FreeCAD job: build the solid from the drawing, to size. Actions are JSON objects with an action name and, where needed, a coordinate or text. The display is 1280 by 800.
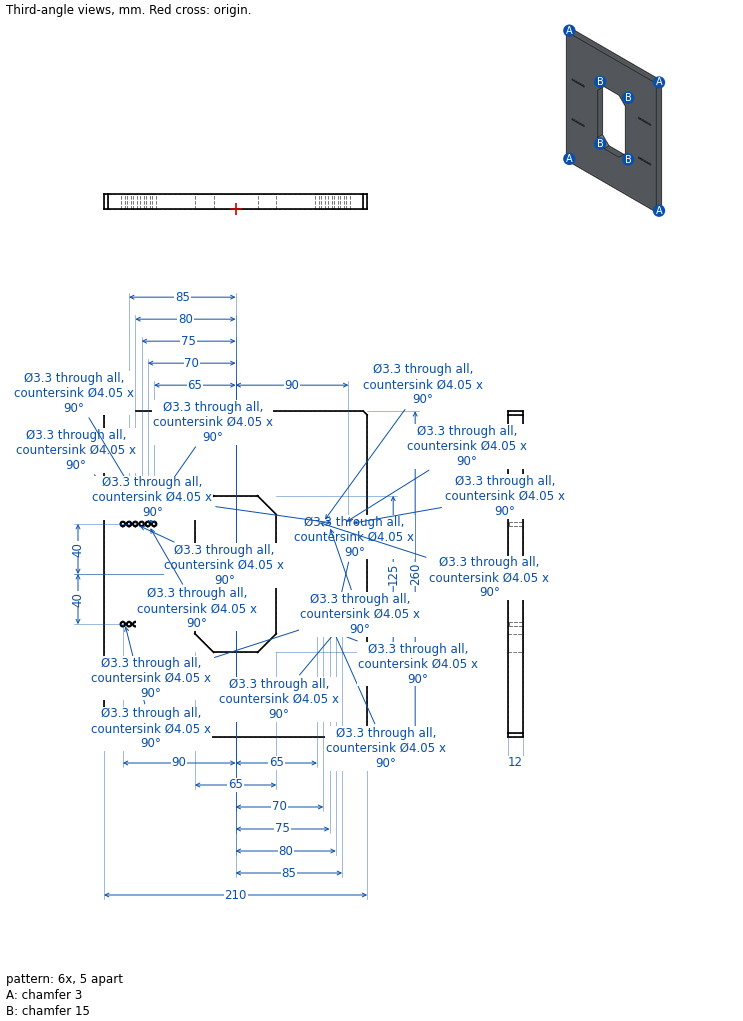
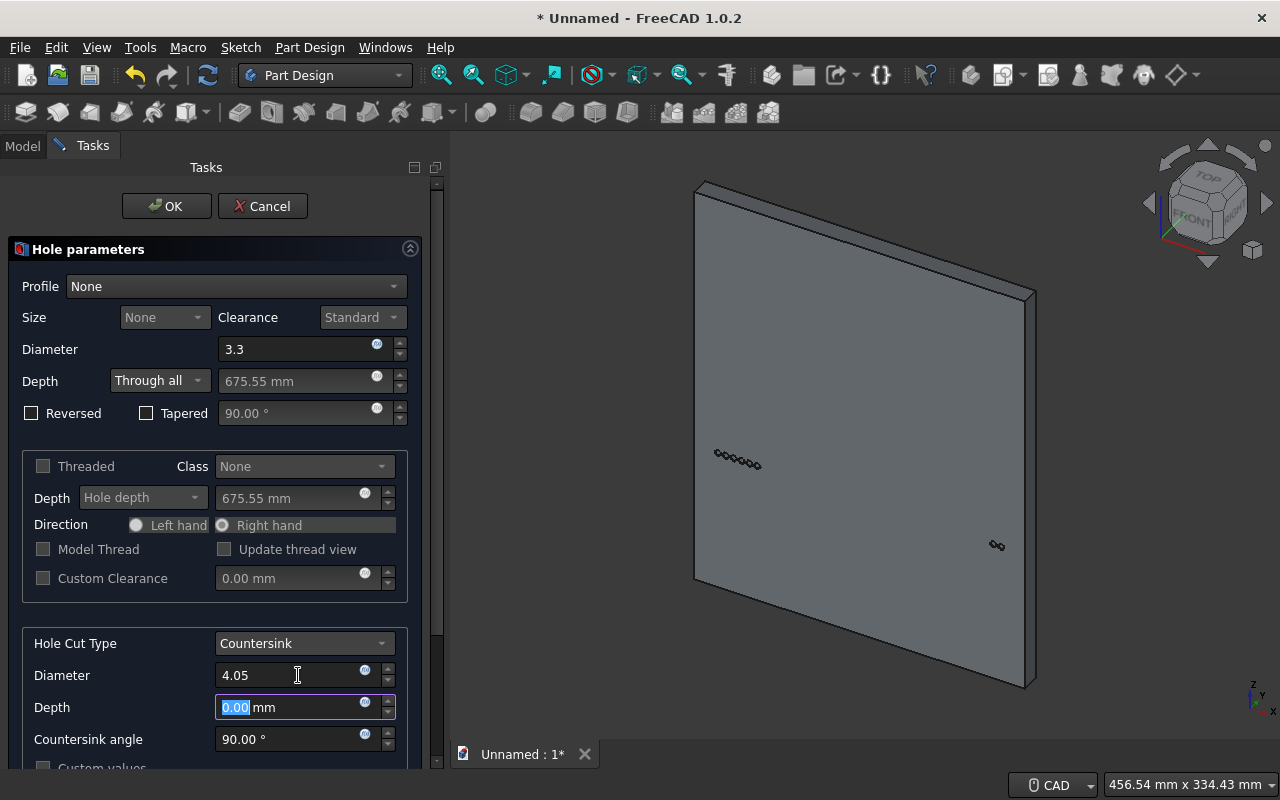
{"action": "left_click", "coordinate": [167, 206]}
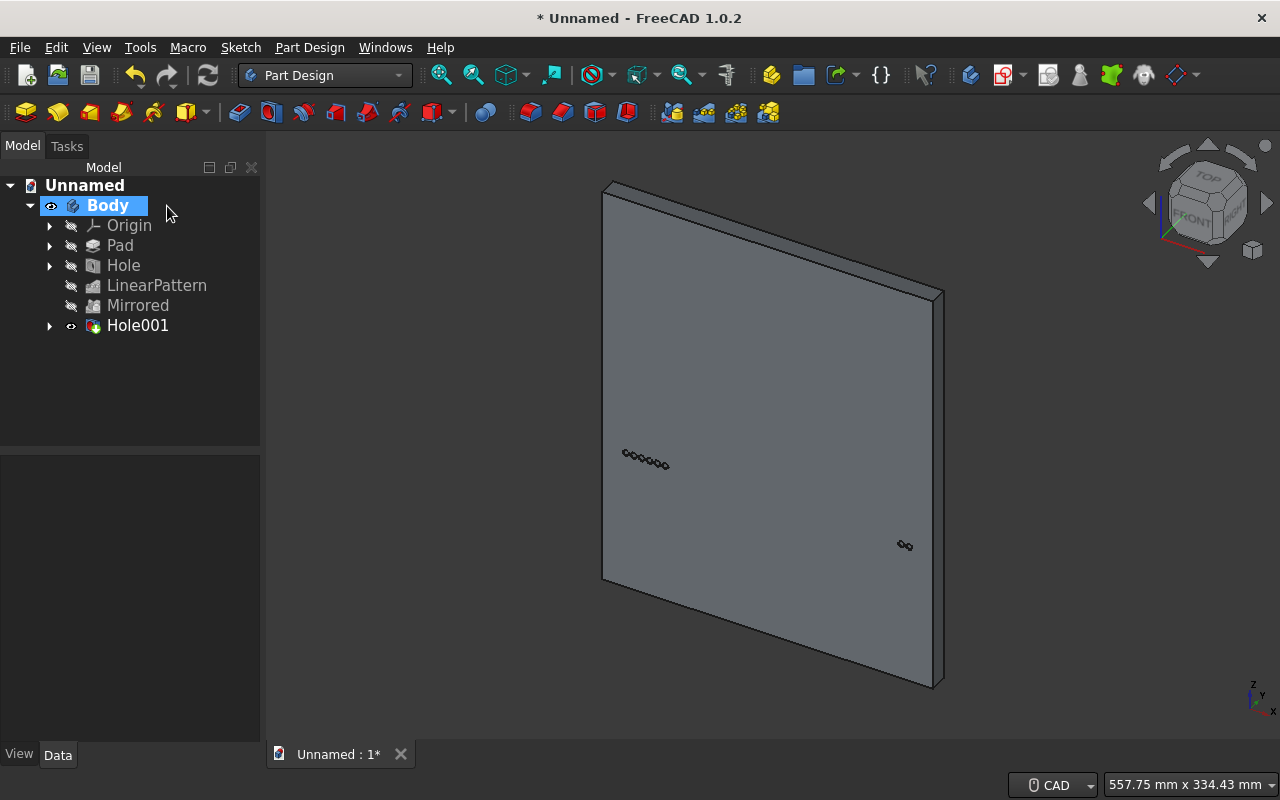
{"action": "left_click", "coordinate": [1004, 76]}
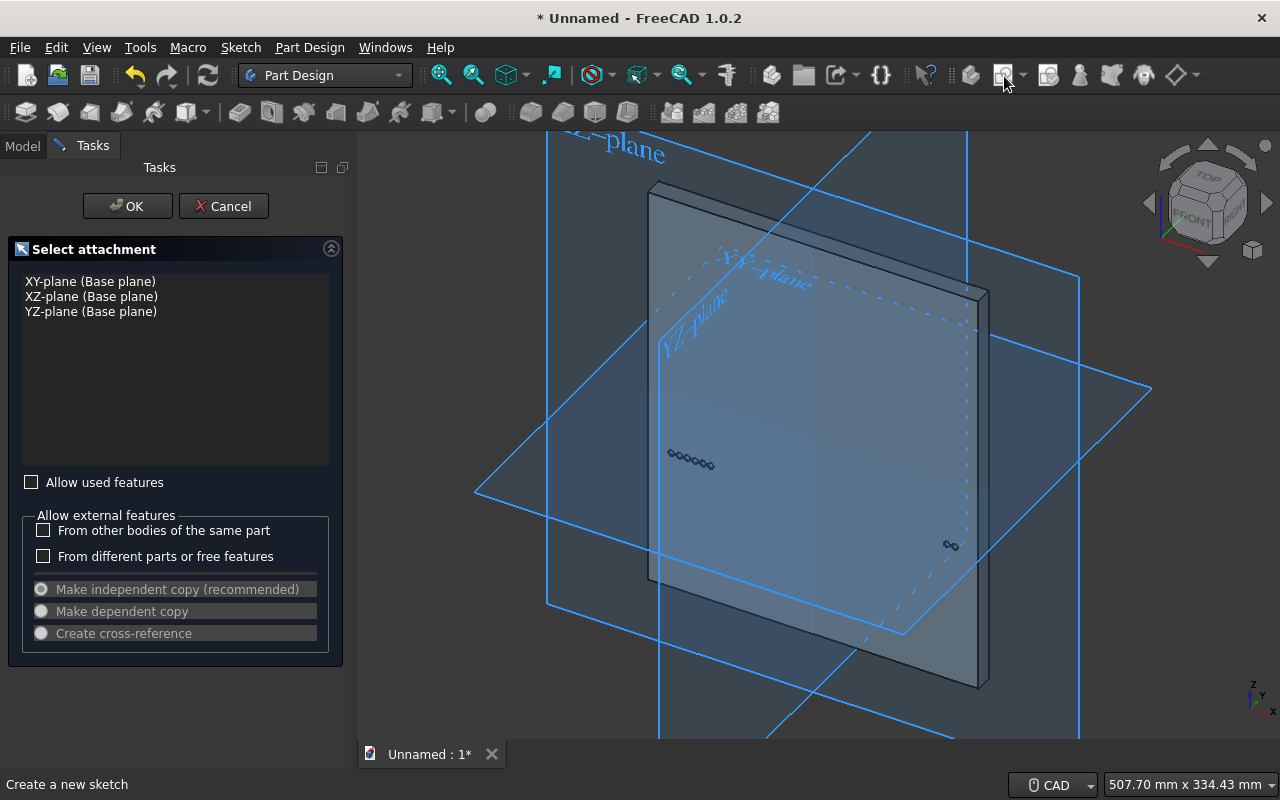
{"action": "left_click", "coordinate": [82, 296]}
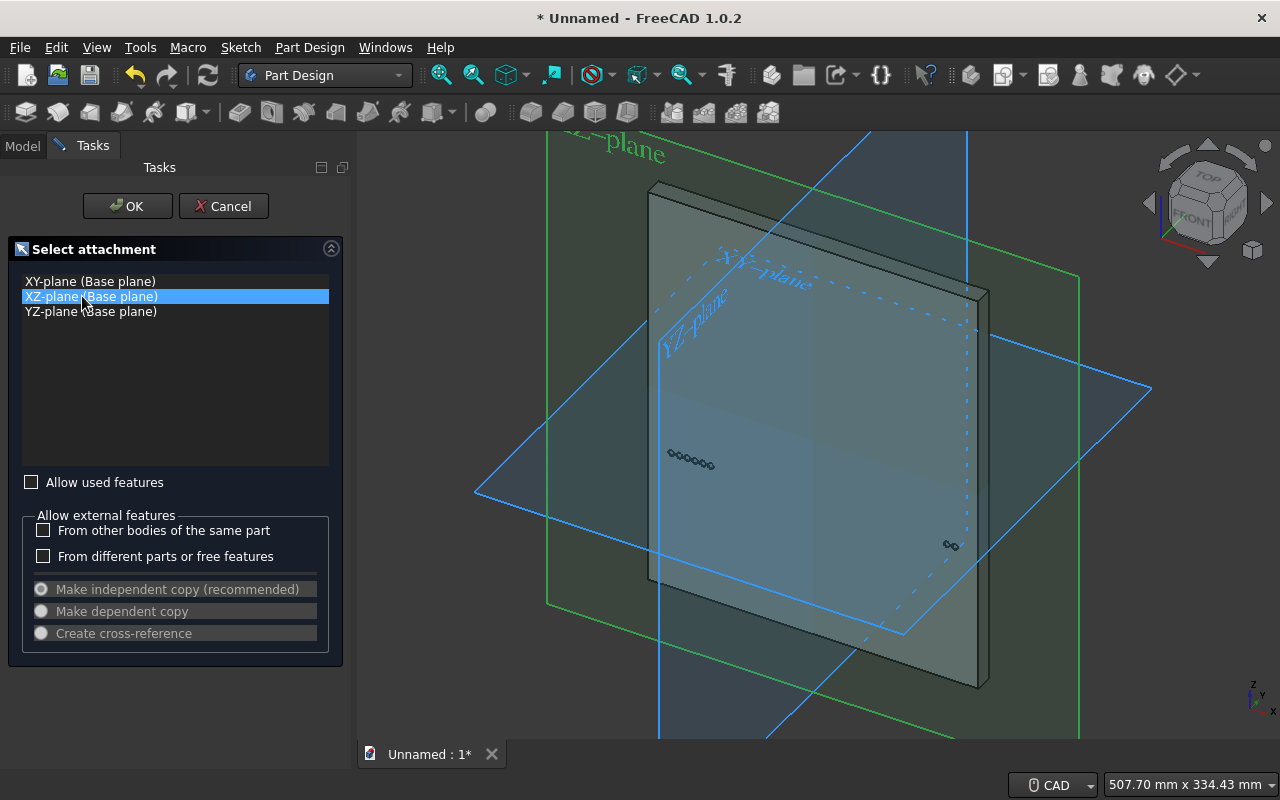
{"action": "left_click", "coordinate": [128, 206]}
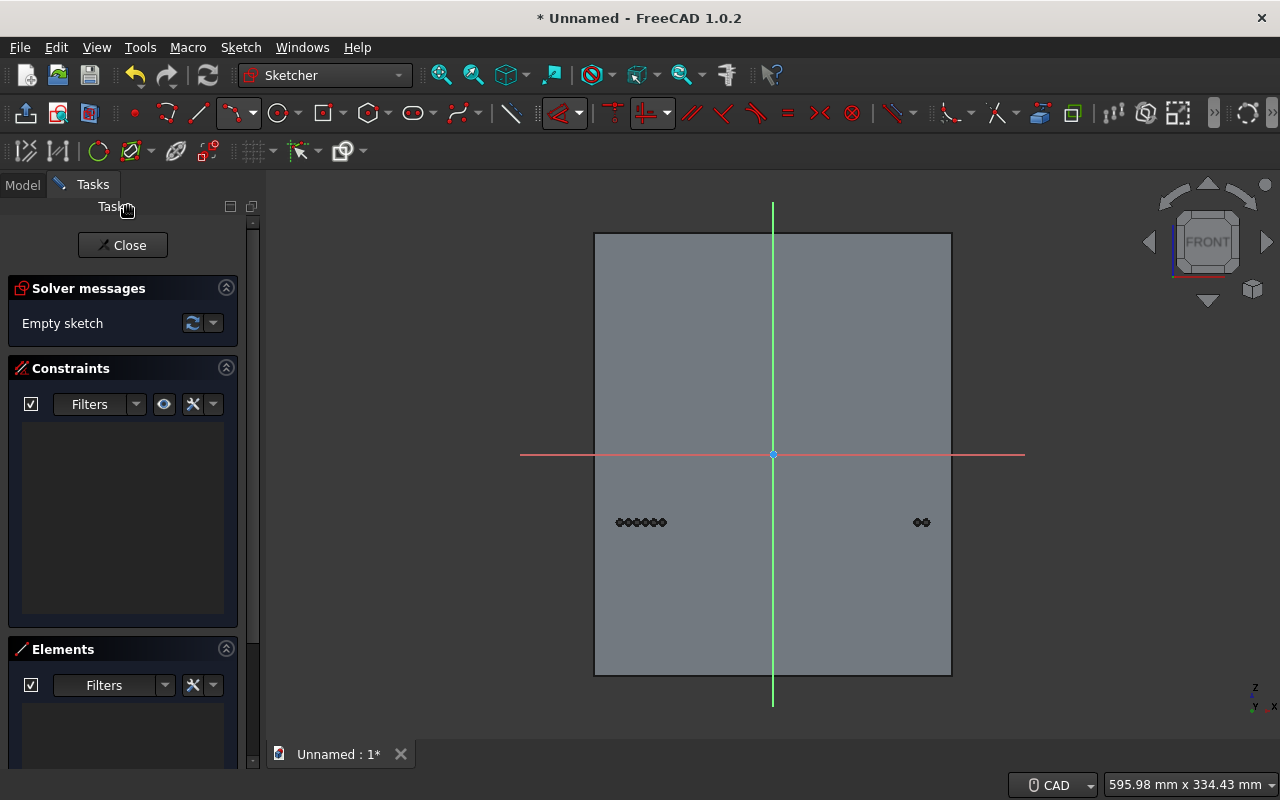
{"action": "scroll", "coordinate": [920, 526], "scroll_direction": "up", "scroll_amount": 15}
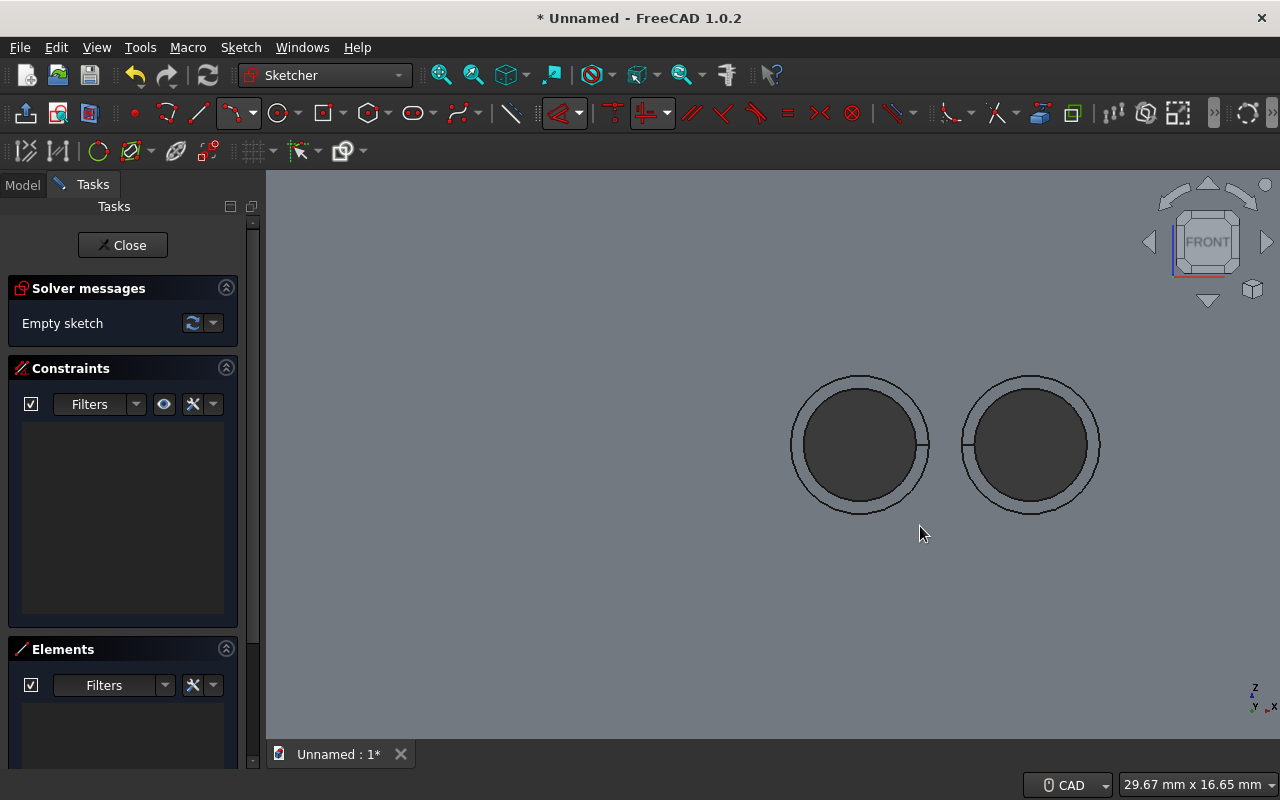
{"action": "scroll", "coordinate": [682, 441], "scroll_direction": "up", "scroll_amount": 6}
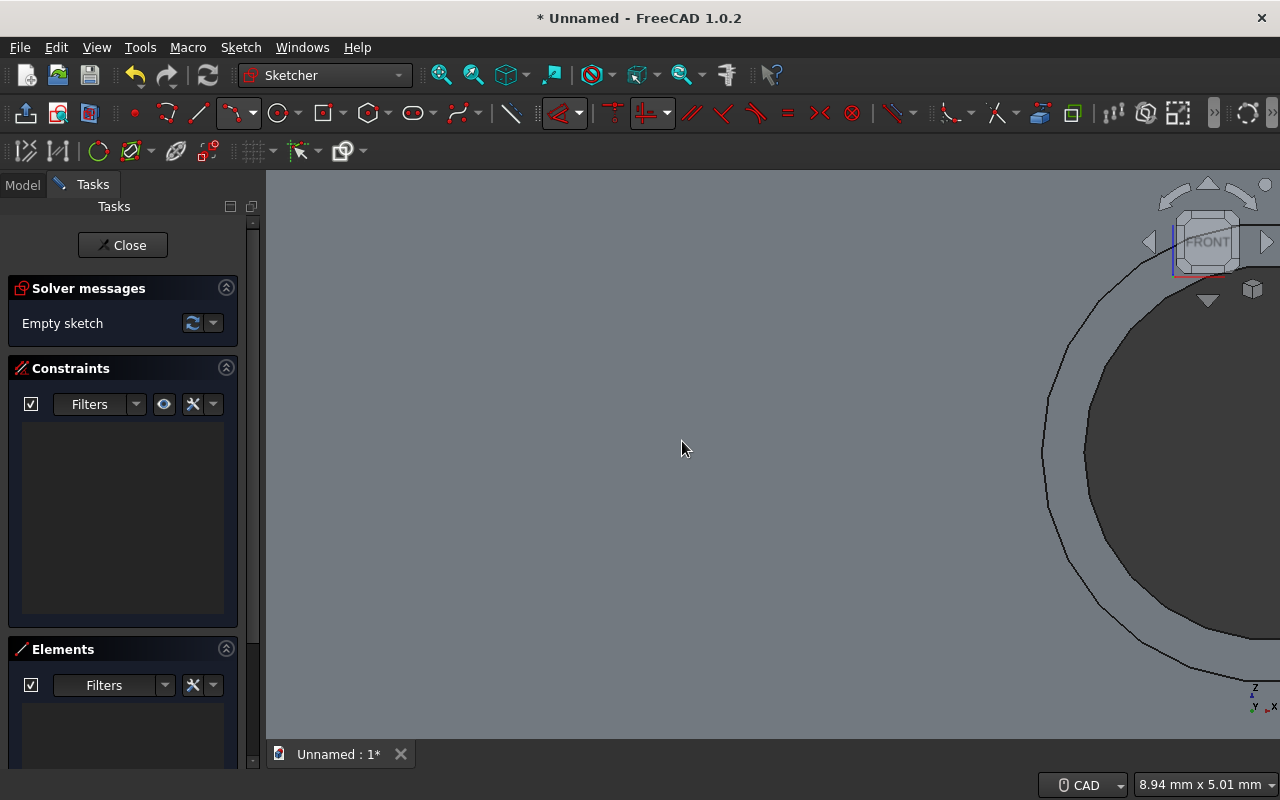
{"action": "left_click", "coordinate": [278, 114]}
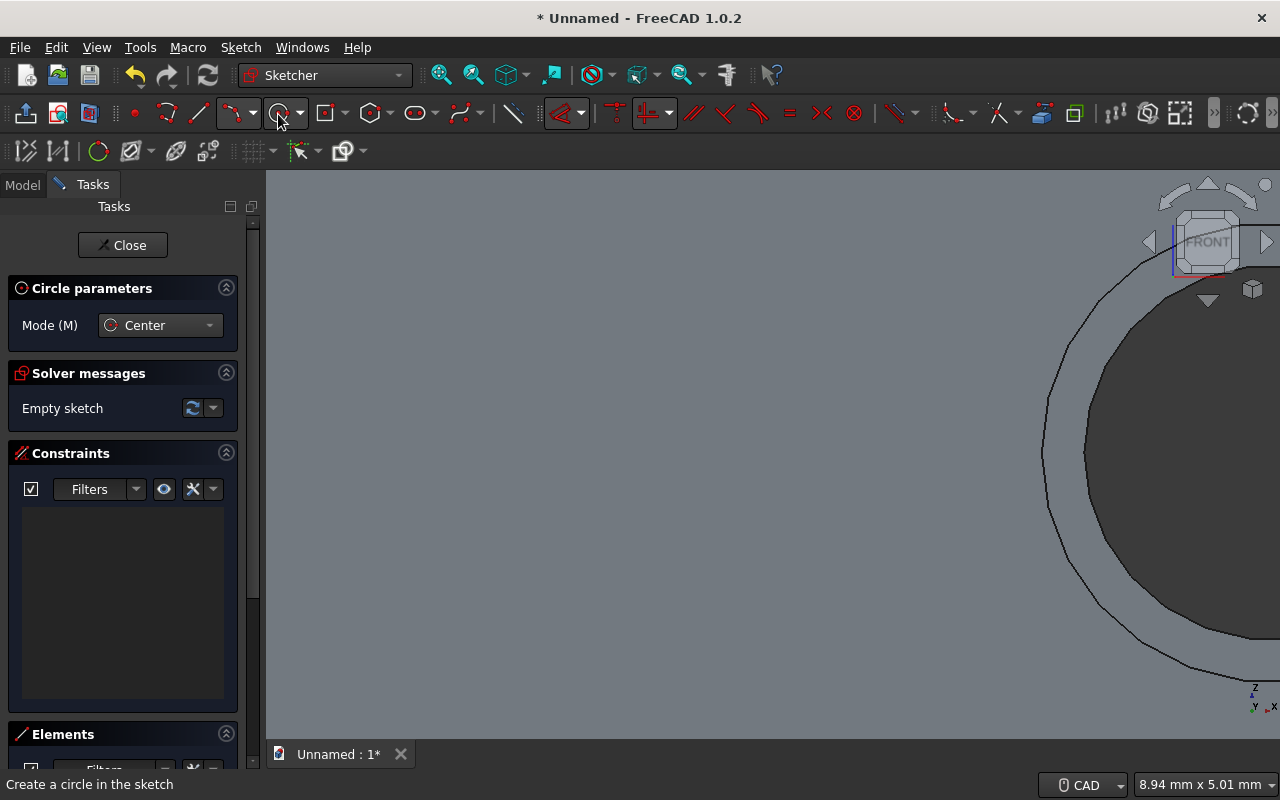
{"action": "left_click", "coordinate": [704, 453]}
{"action": "mouse_move", "coordinate": [837, 320]}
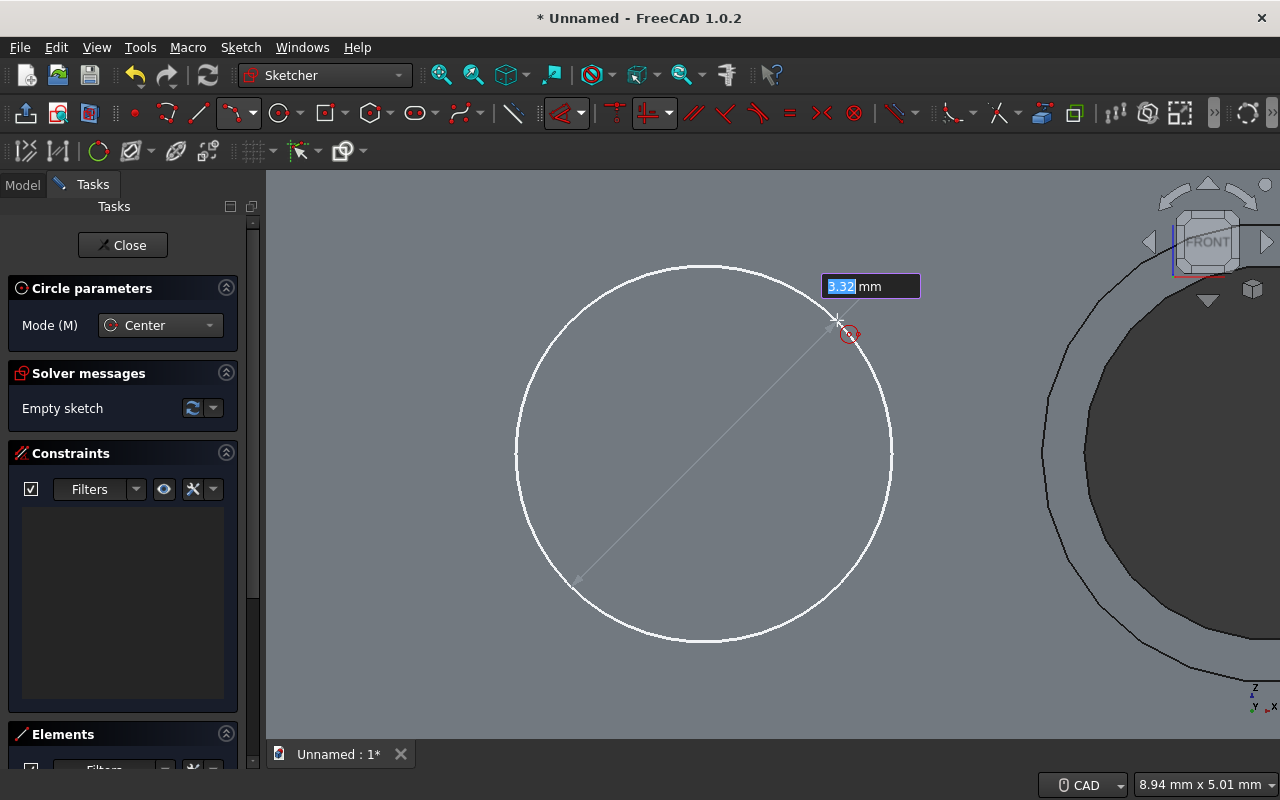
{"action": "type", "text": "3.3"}
{"action": "key", "text": "Return"}
{"action": "key", "text": "Escape"}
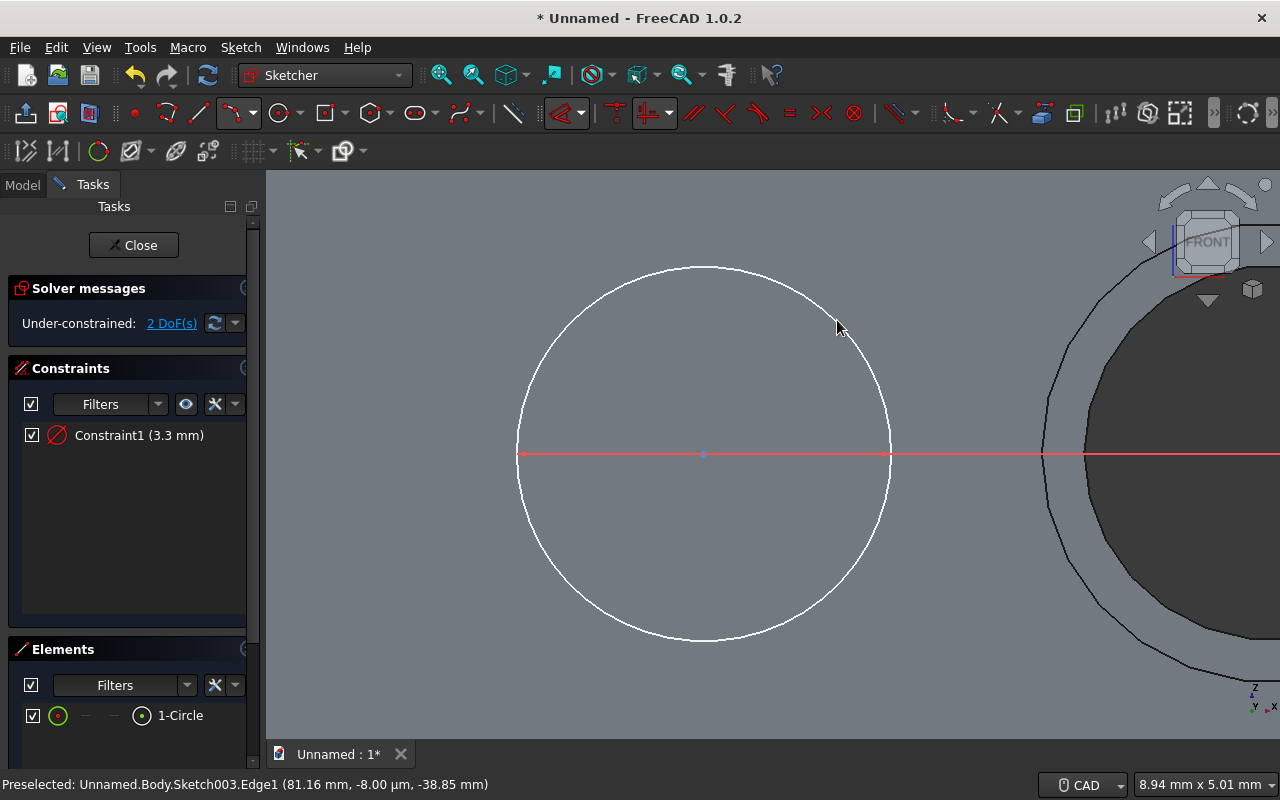
{"action": "left_click", "coordinate": [704, 454]}